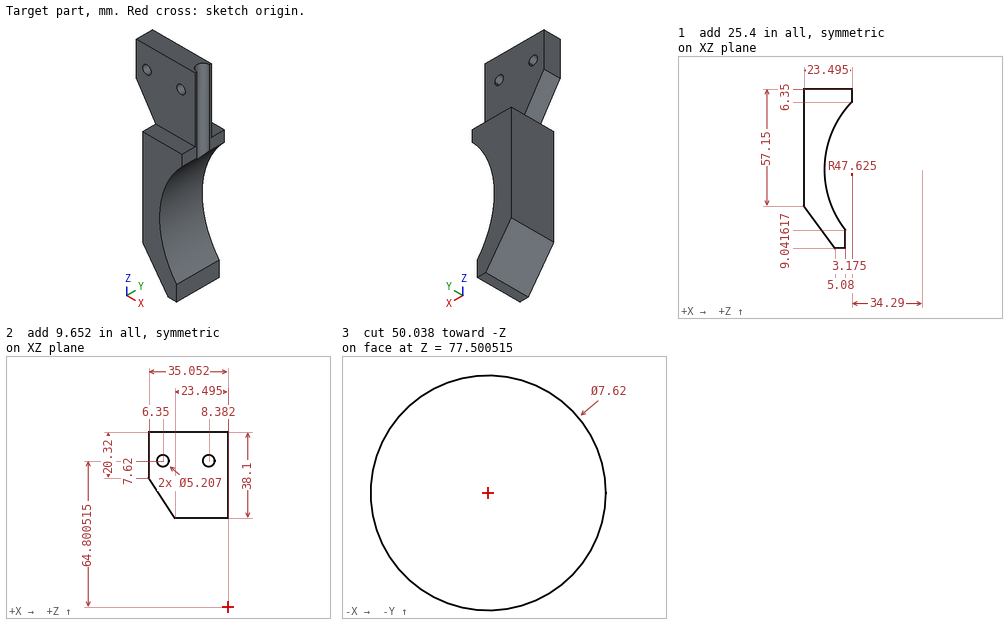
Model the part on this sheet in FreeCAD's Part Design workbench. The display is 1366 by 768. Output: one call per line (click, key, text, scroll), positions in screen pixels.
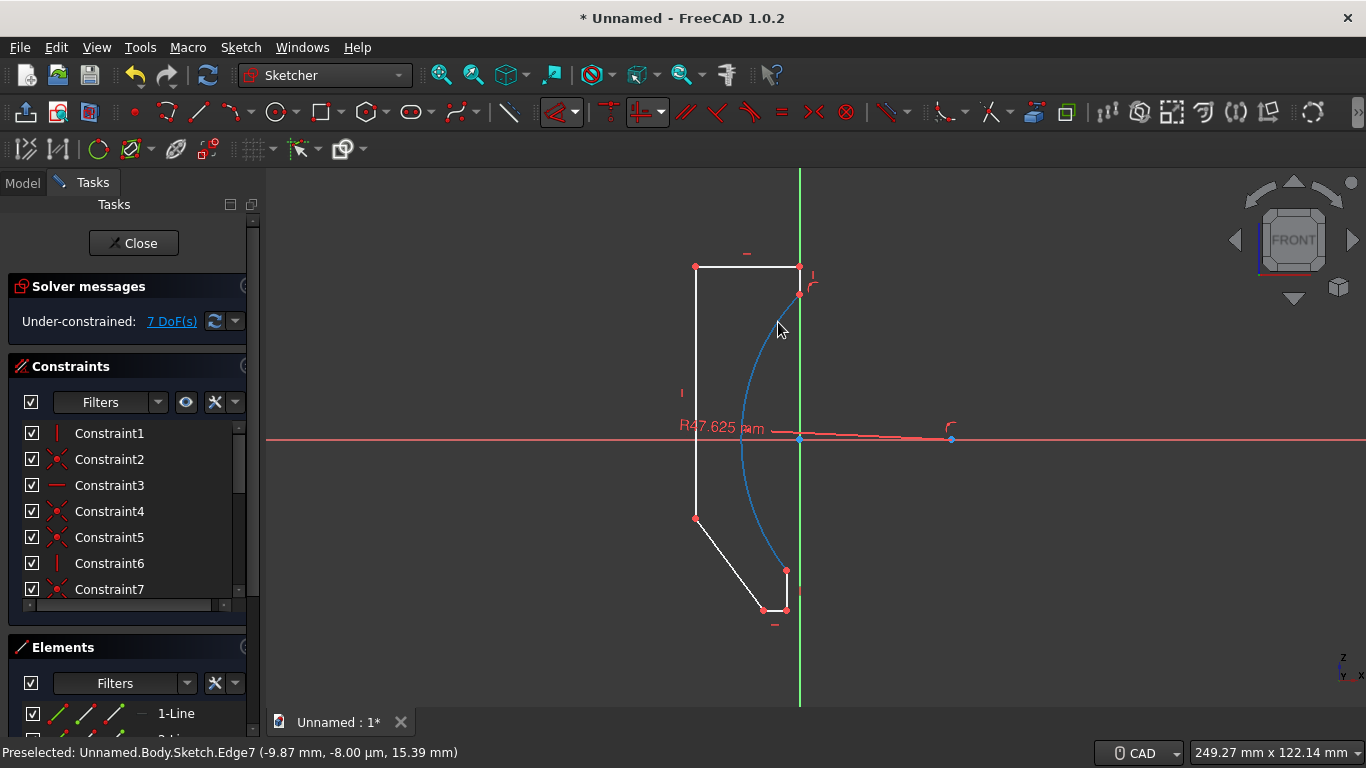
scroll(780, 611, up, 4)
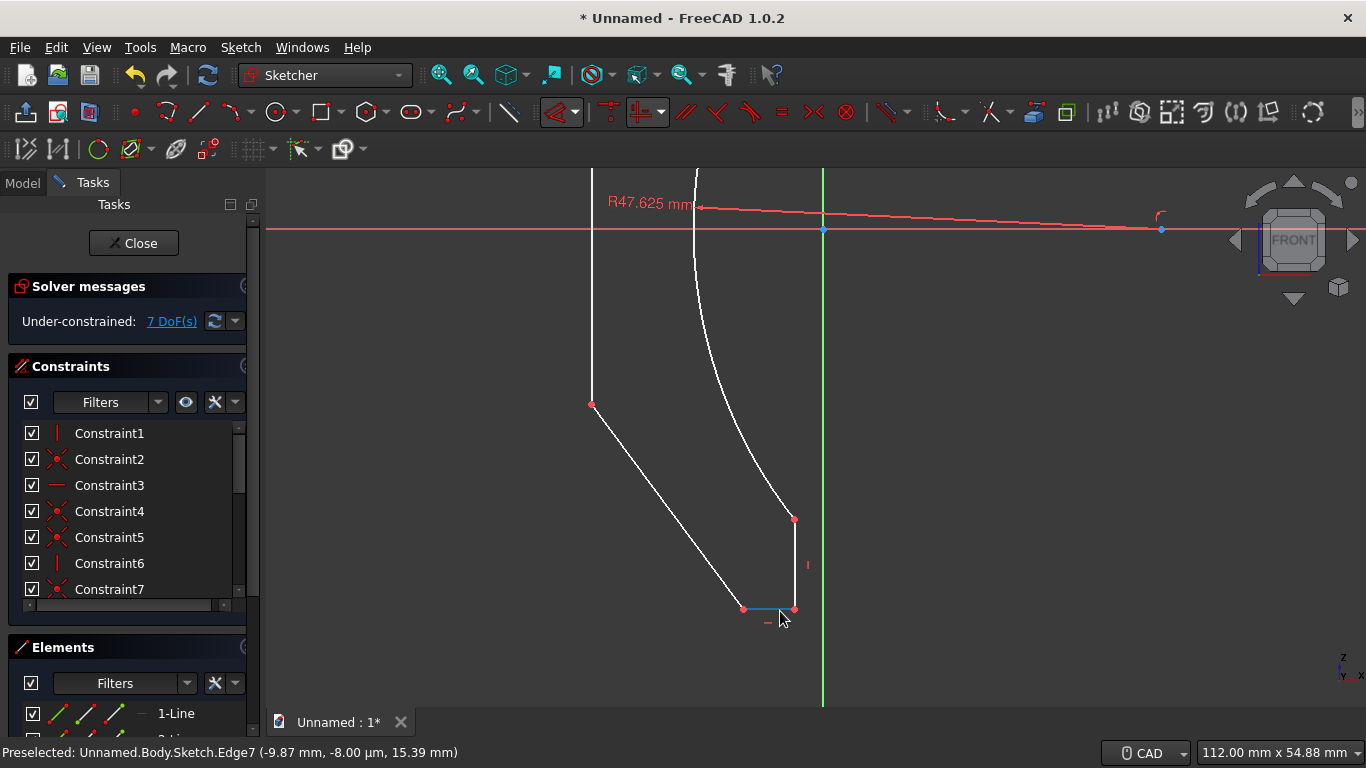
click(779, 609)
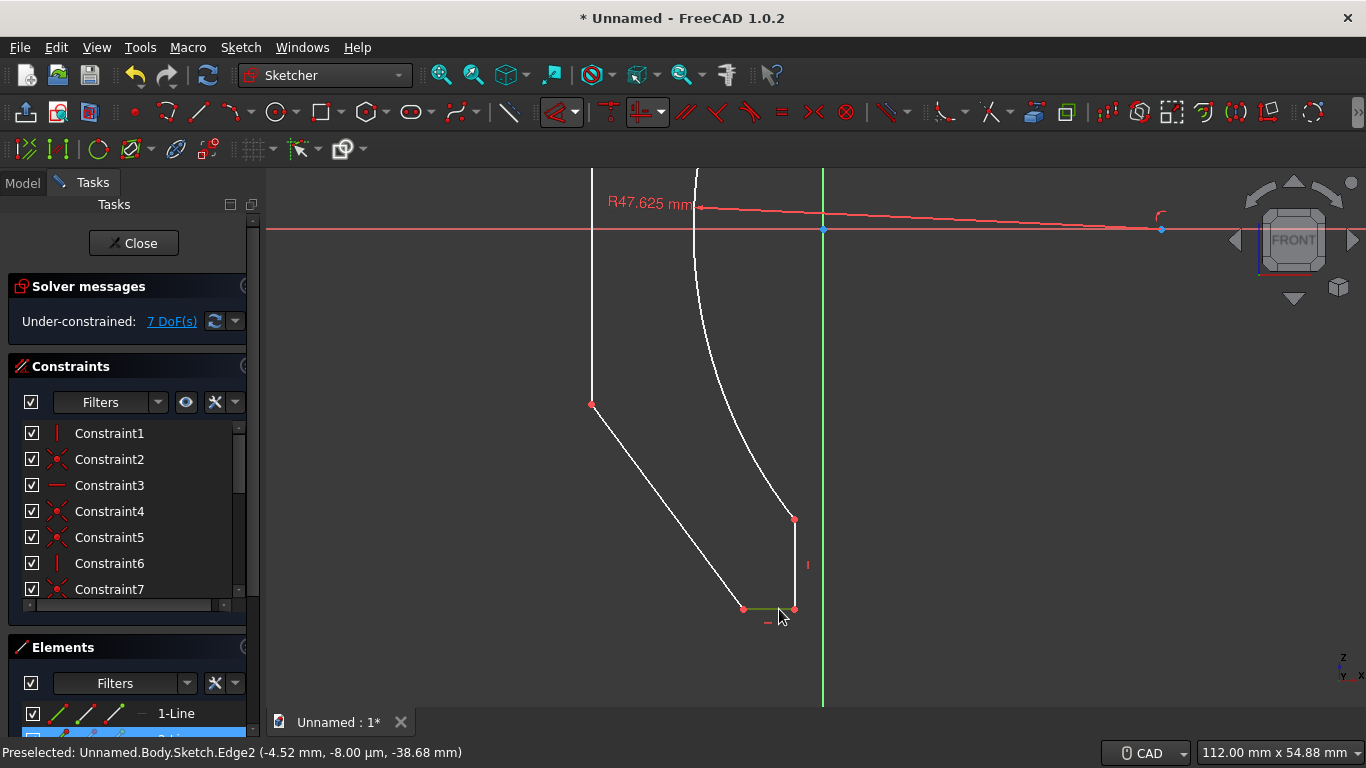
key(l)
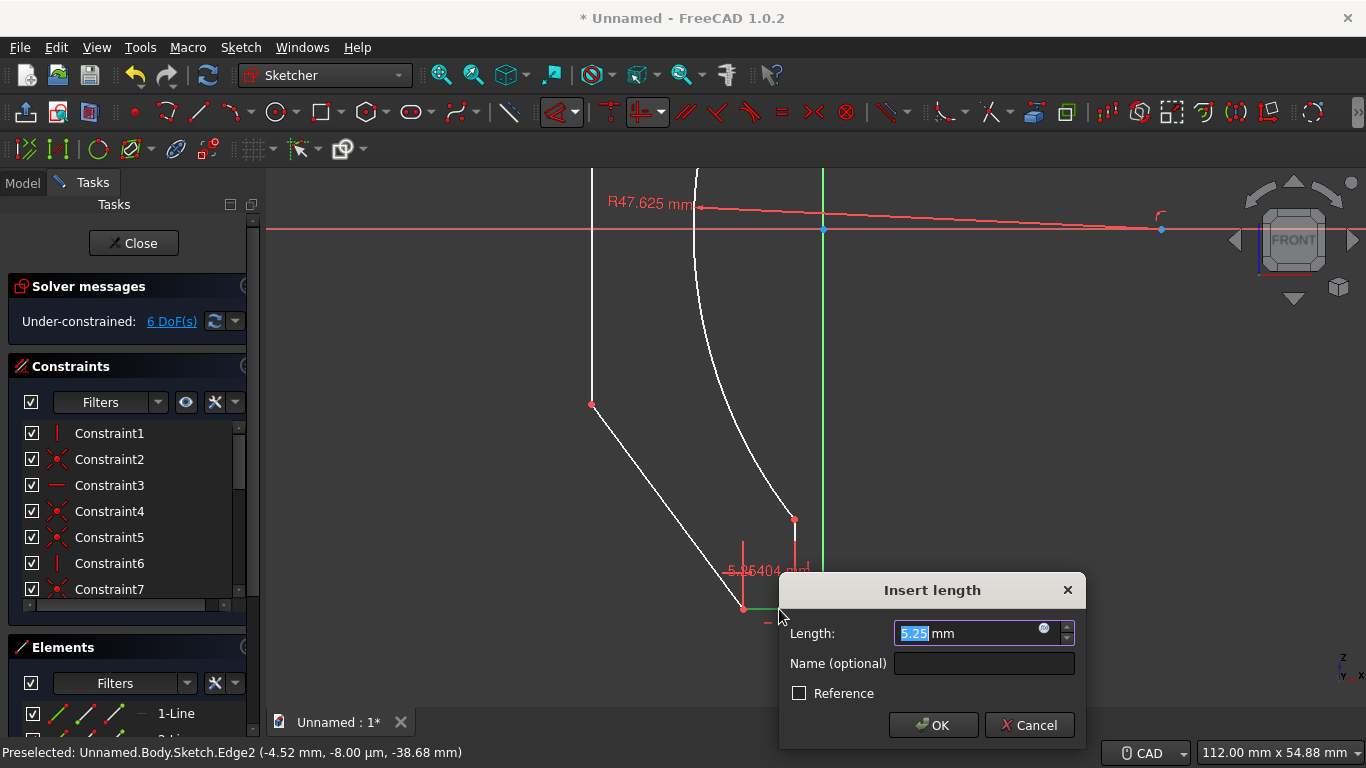
text(5.08)
key(Return)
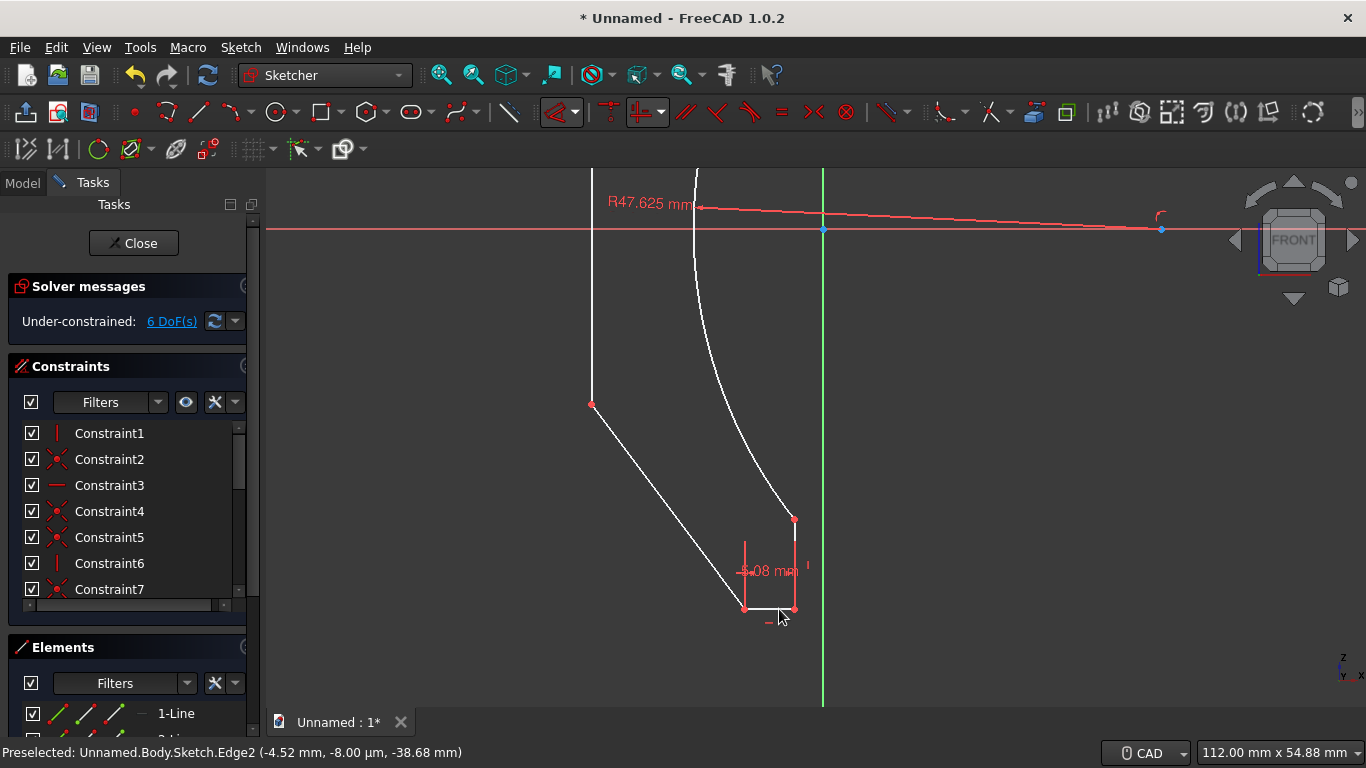
scroll(780, 611, down, 4)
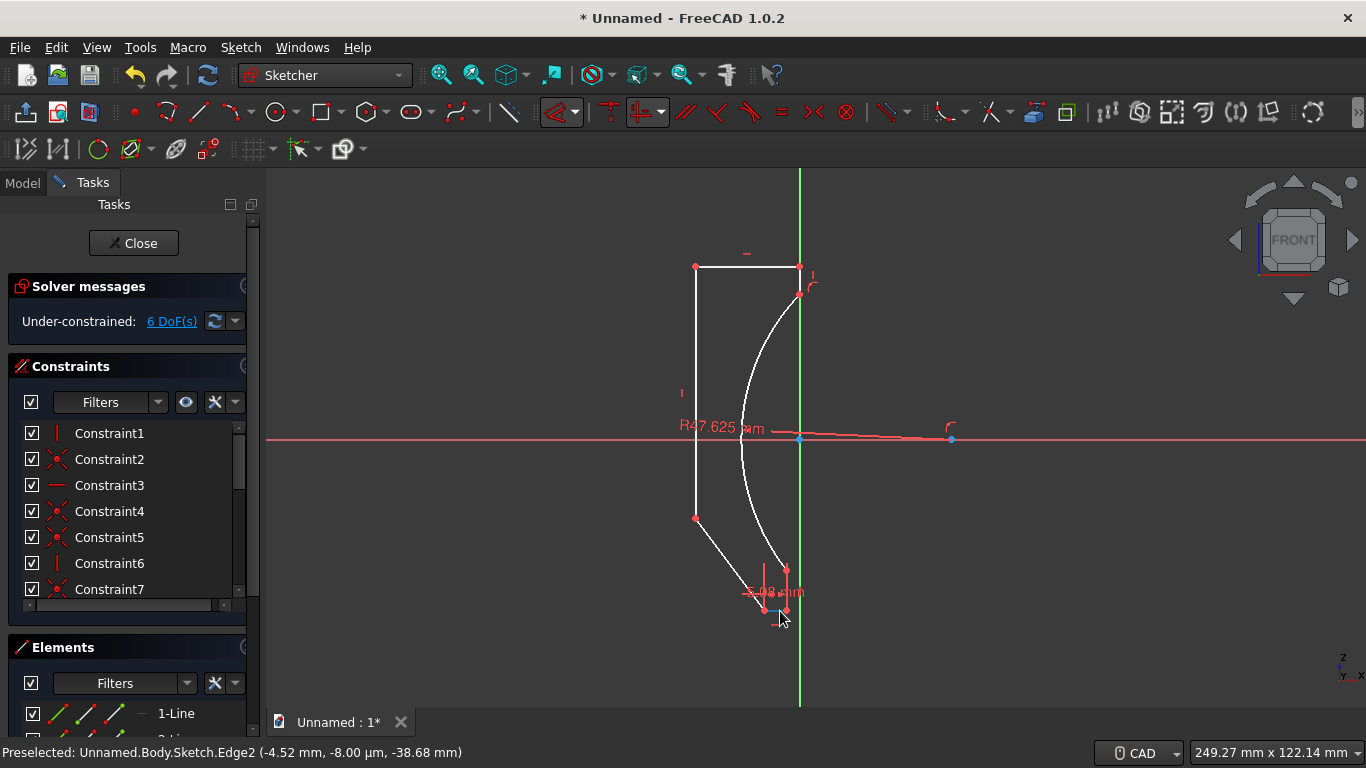
scroll(800, 275, up, 3)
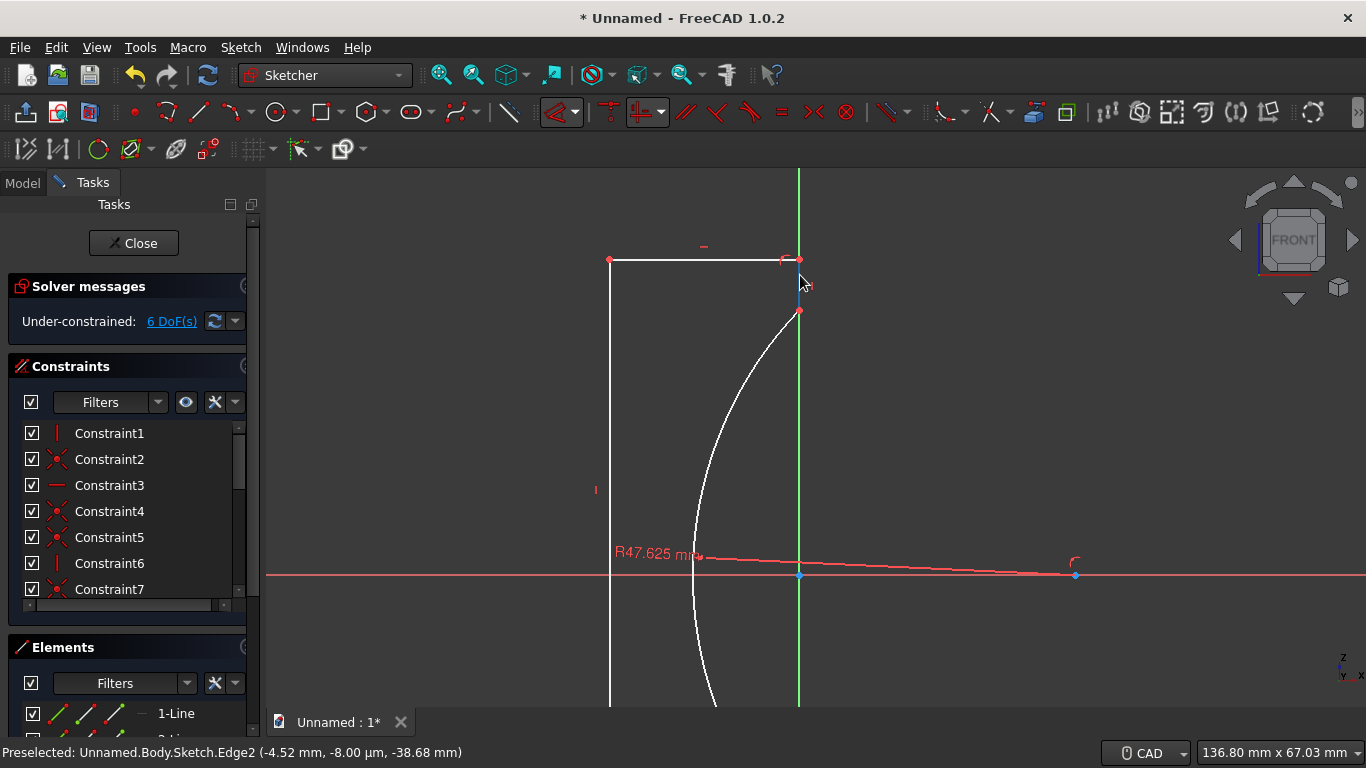
click(799, 275)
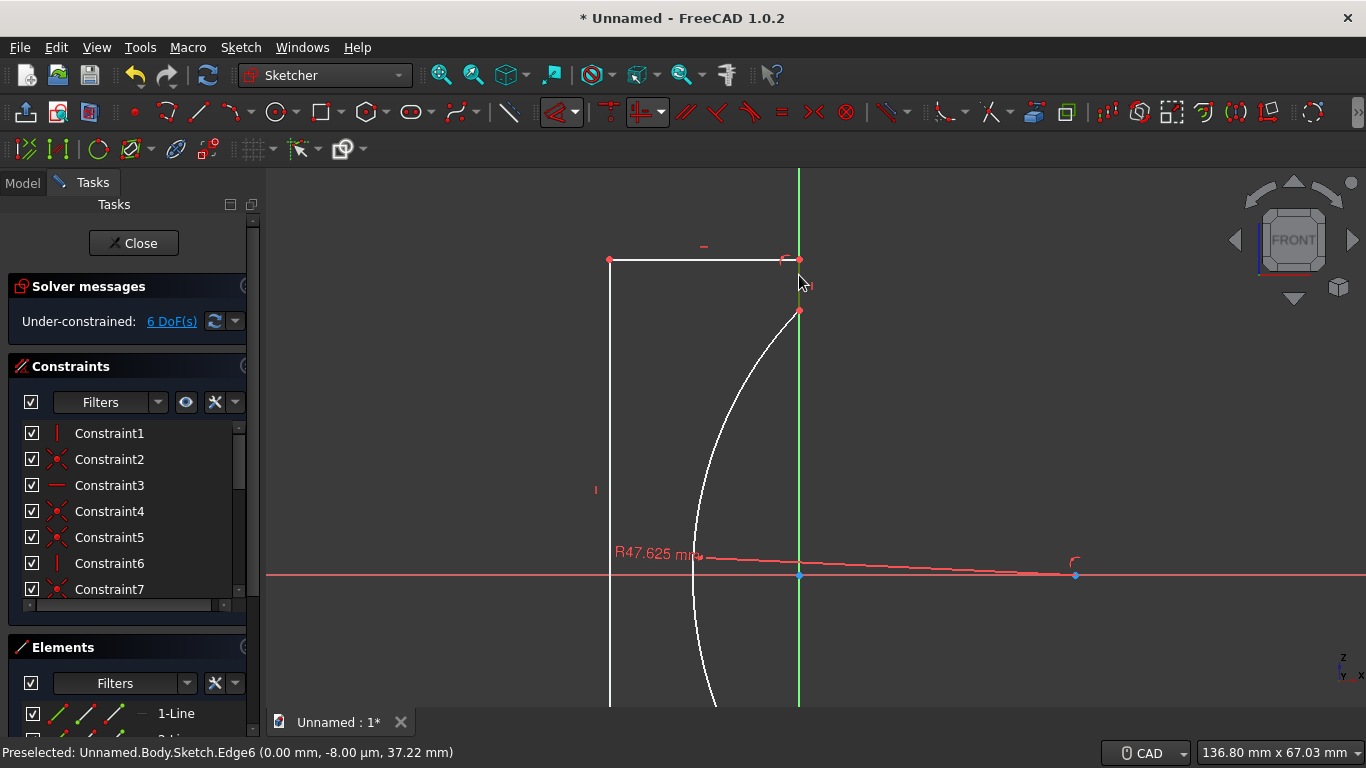
click(578, 112)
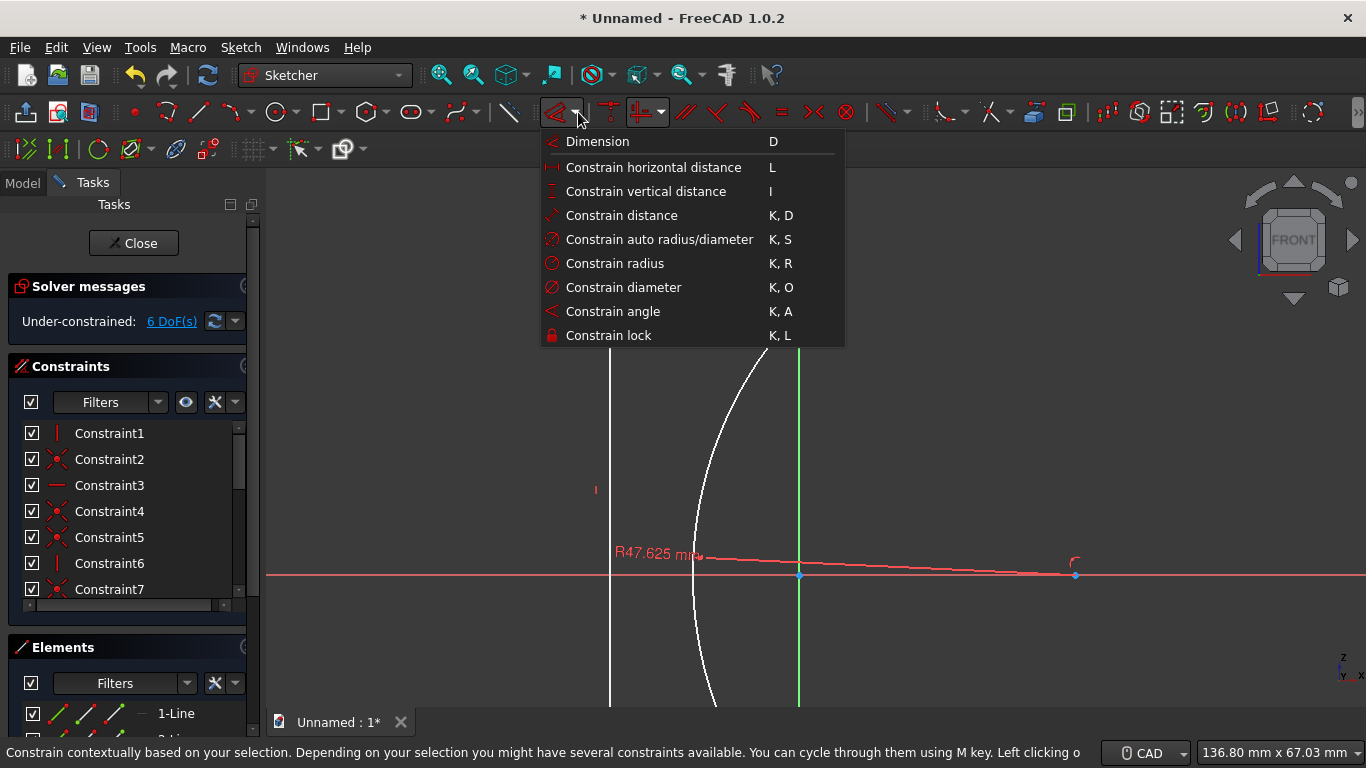
click(693, 191)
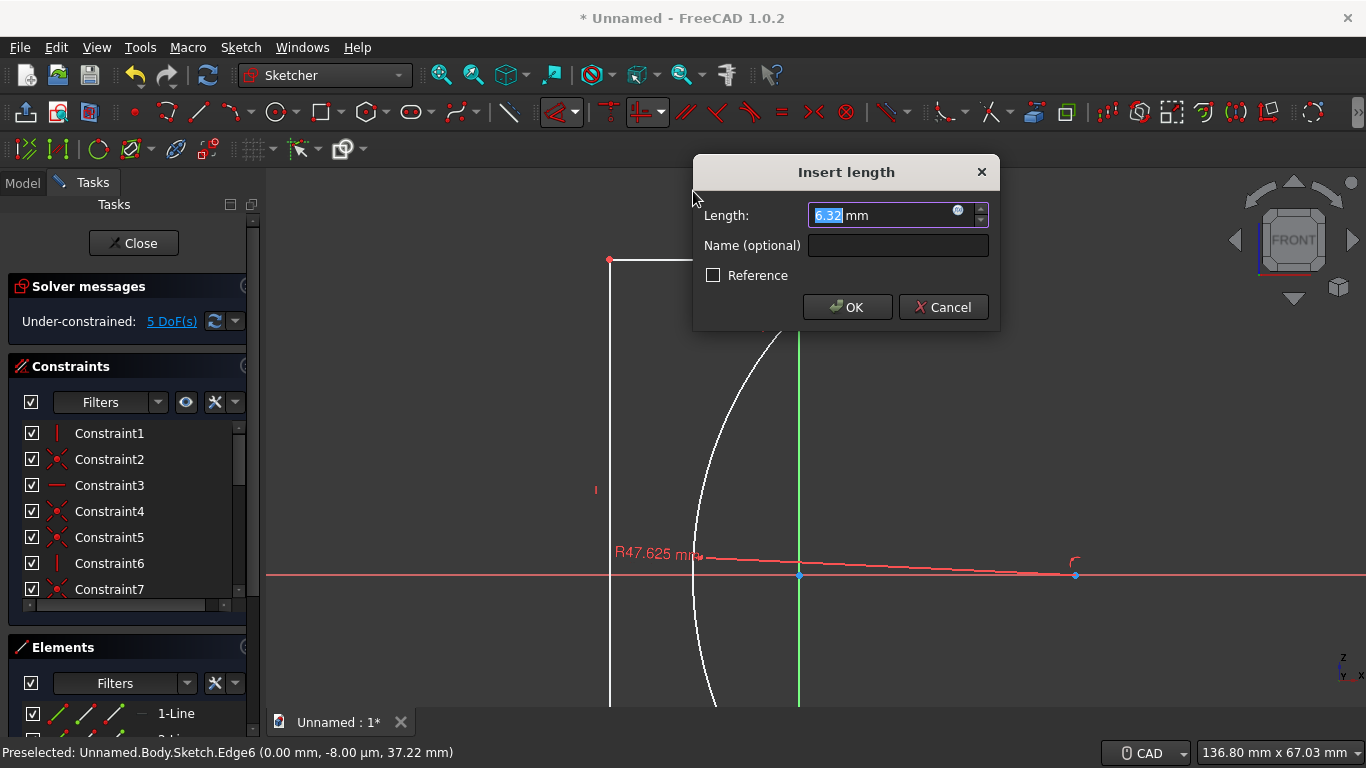
text(6.35)
key(Return)